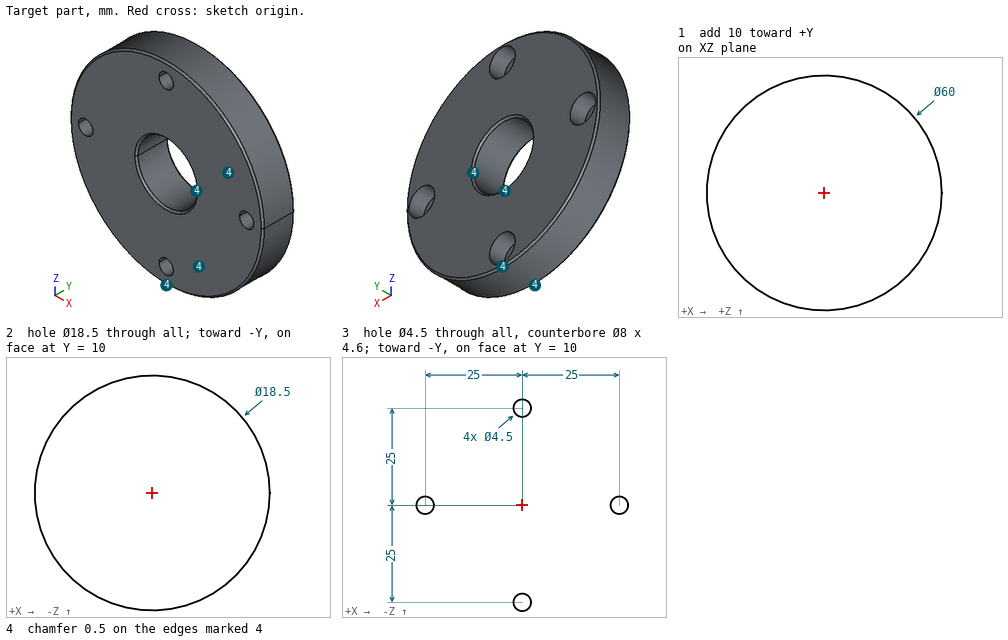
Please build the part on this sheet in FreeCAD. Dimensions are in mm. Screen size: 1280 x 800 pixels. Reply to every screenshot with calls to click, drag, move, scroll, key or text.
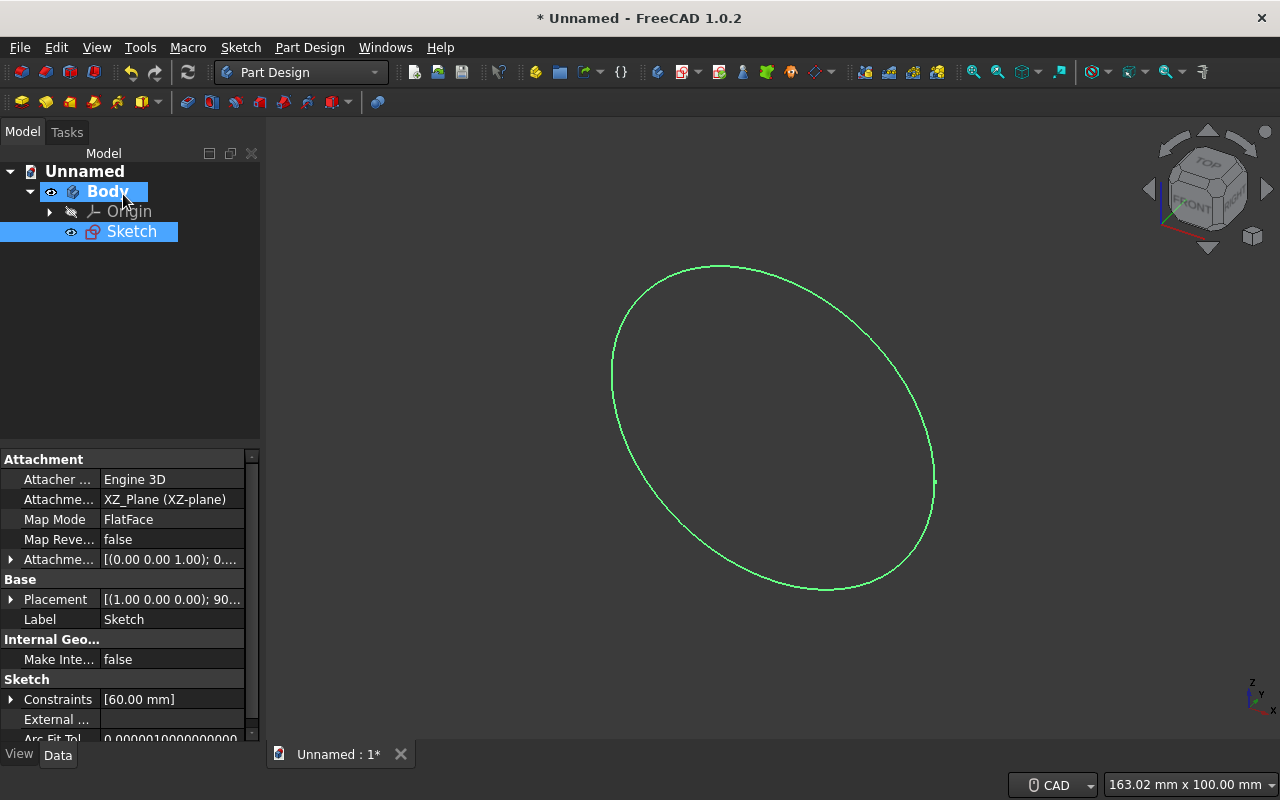
click(22, 102)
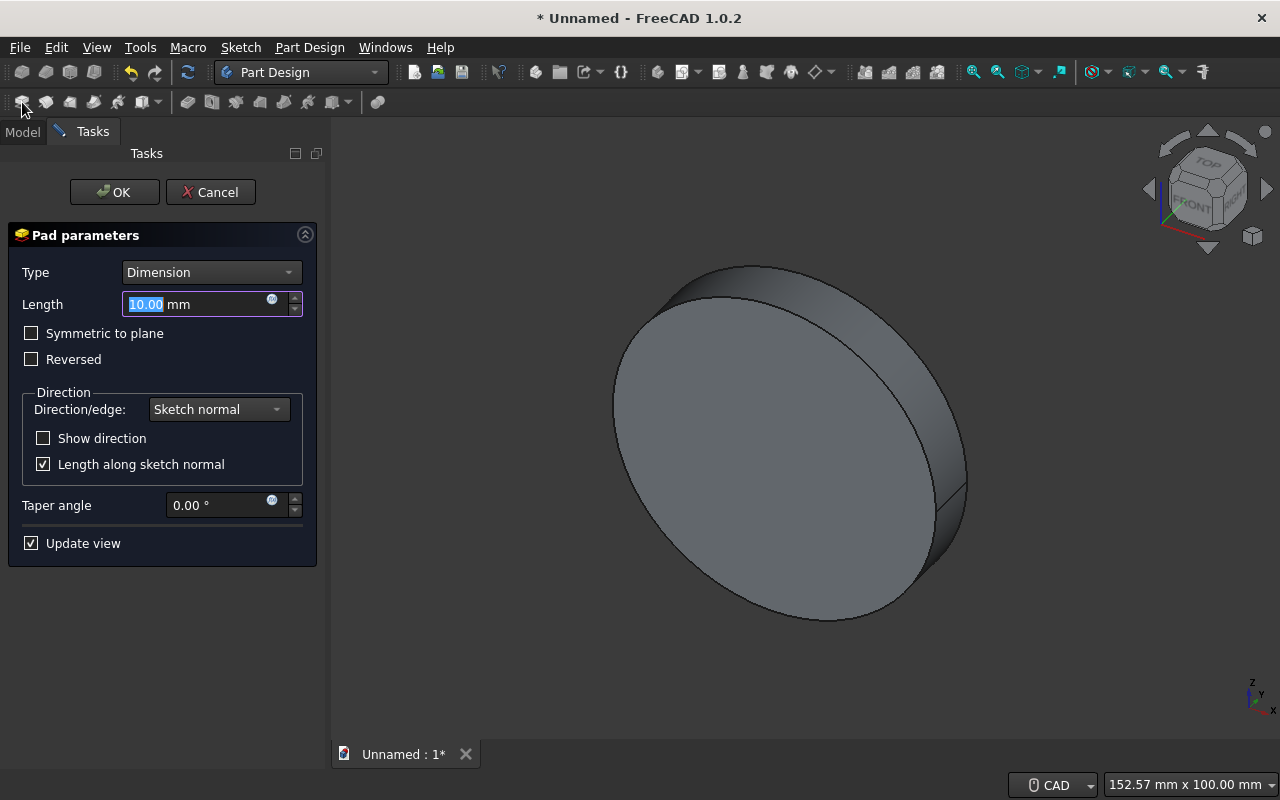
text(10)
key(Tab)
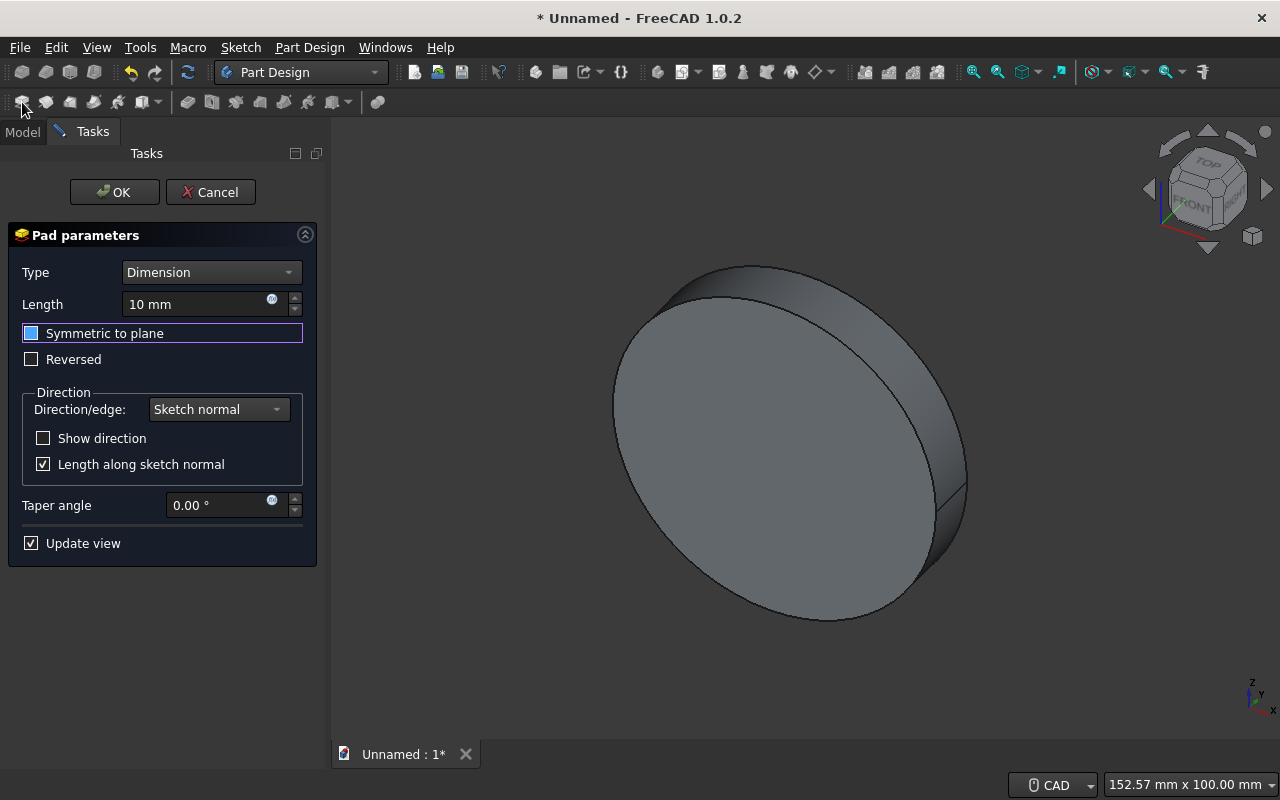
click(30, 359)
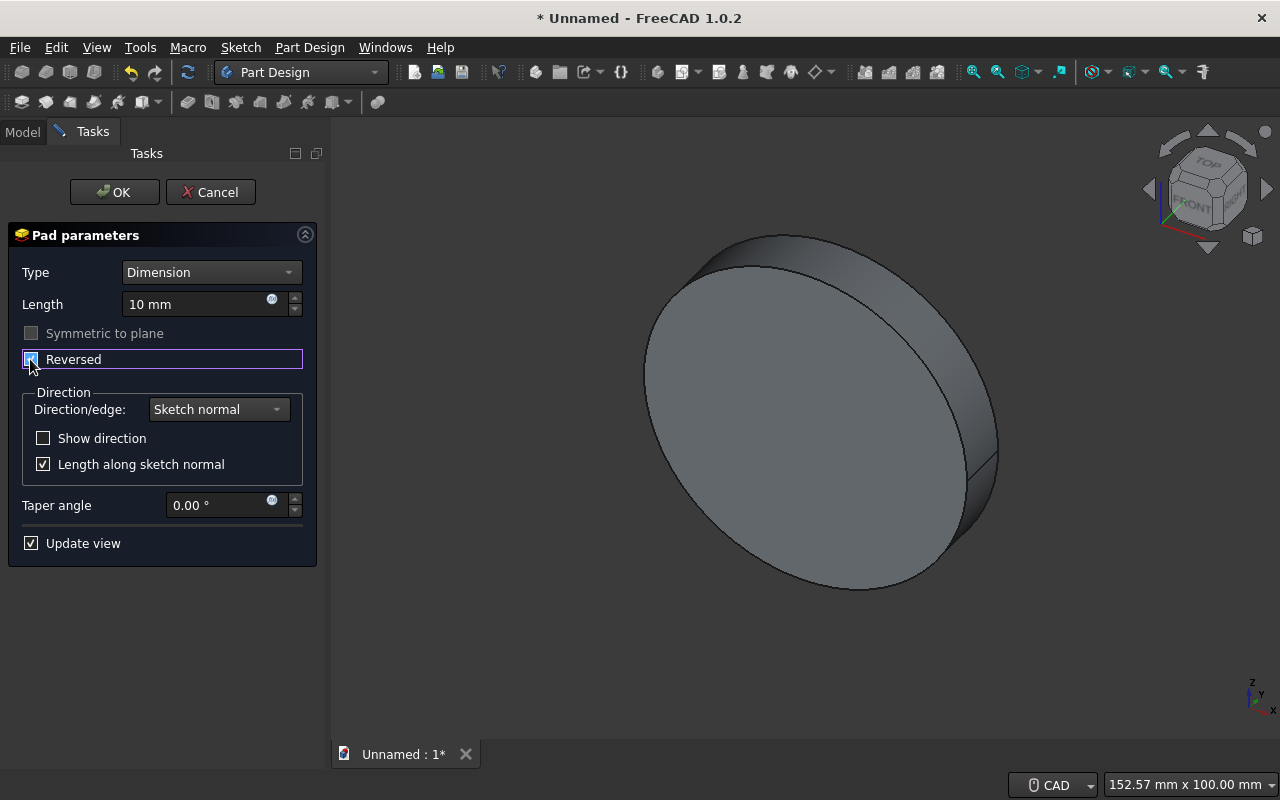
click(115, 192)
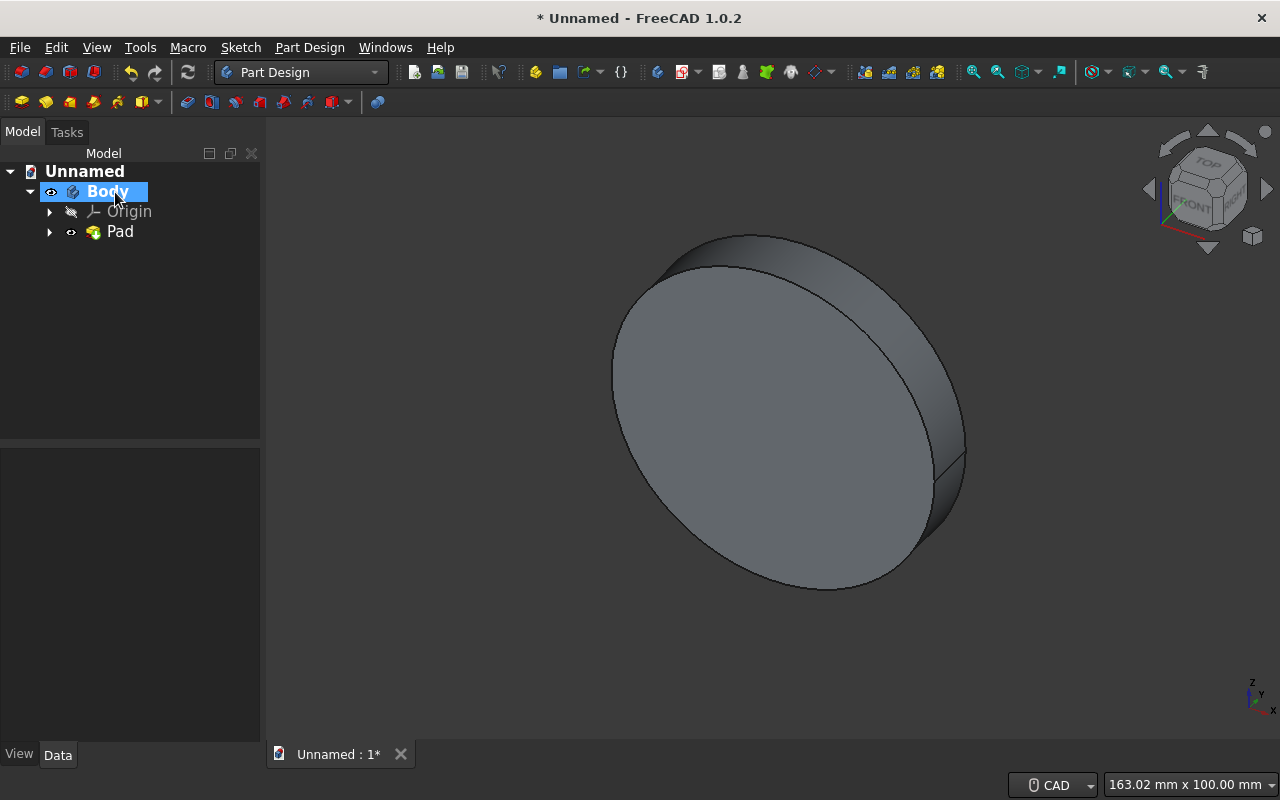
key(4)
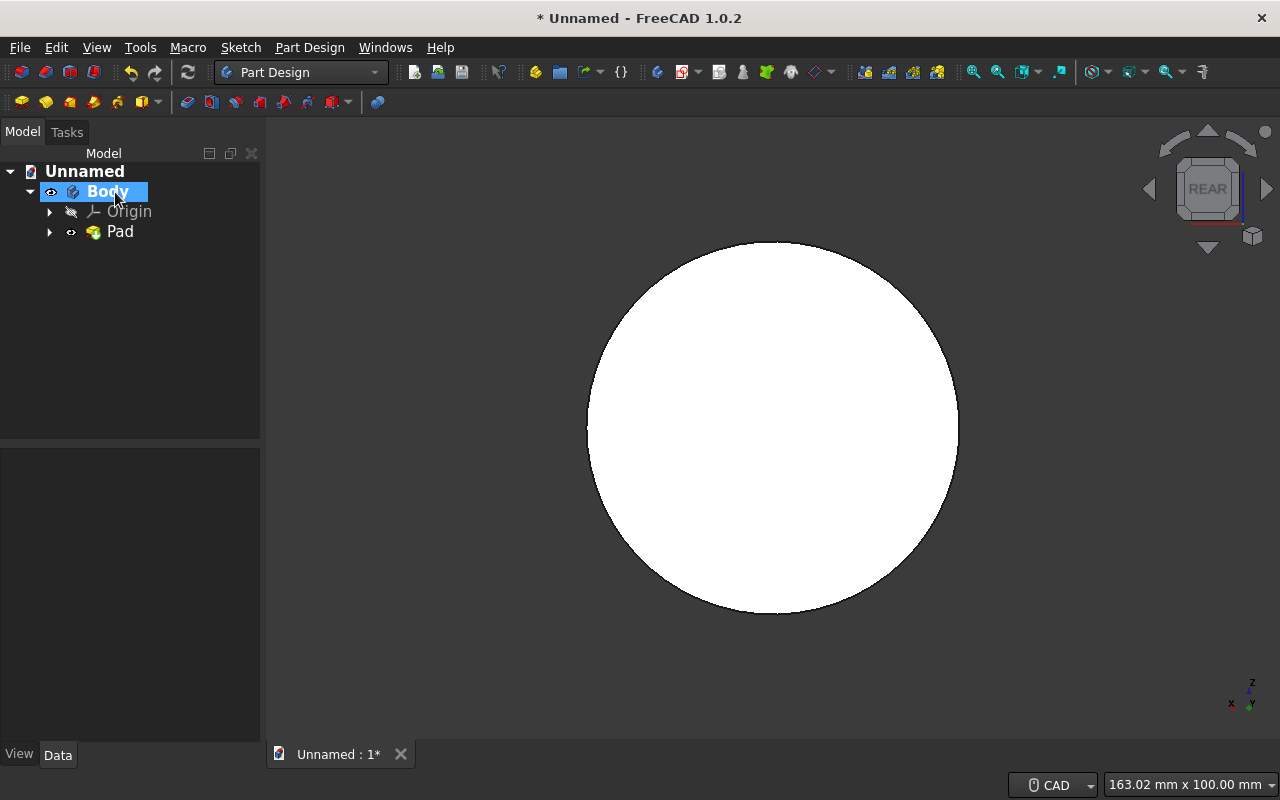
click(773, 427)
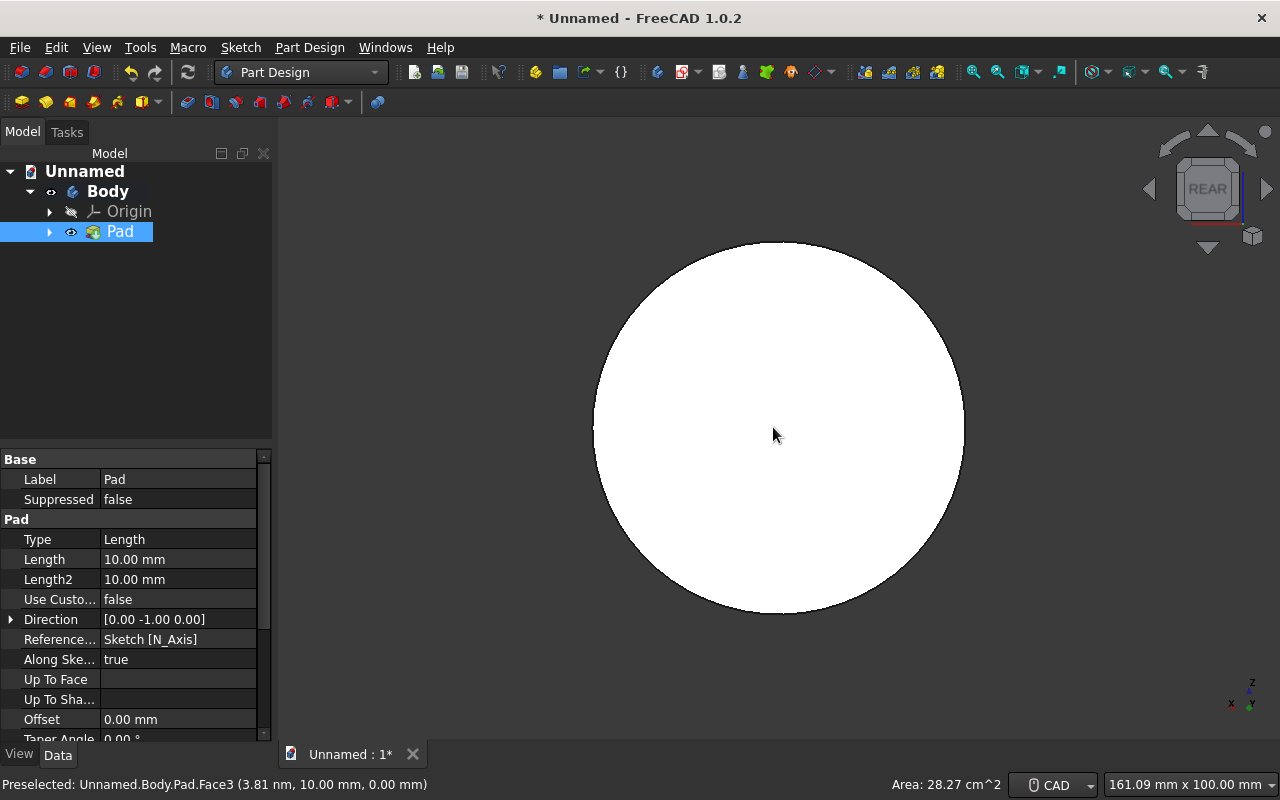
click(682, 72)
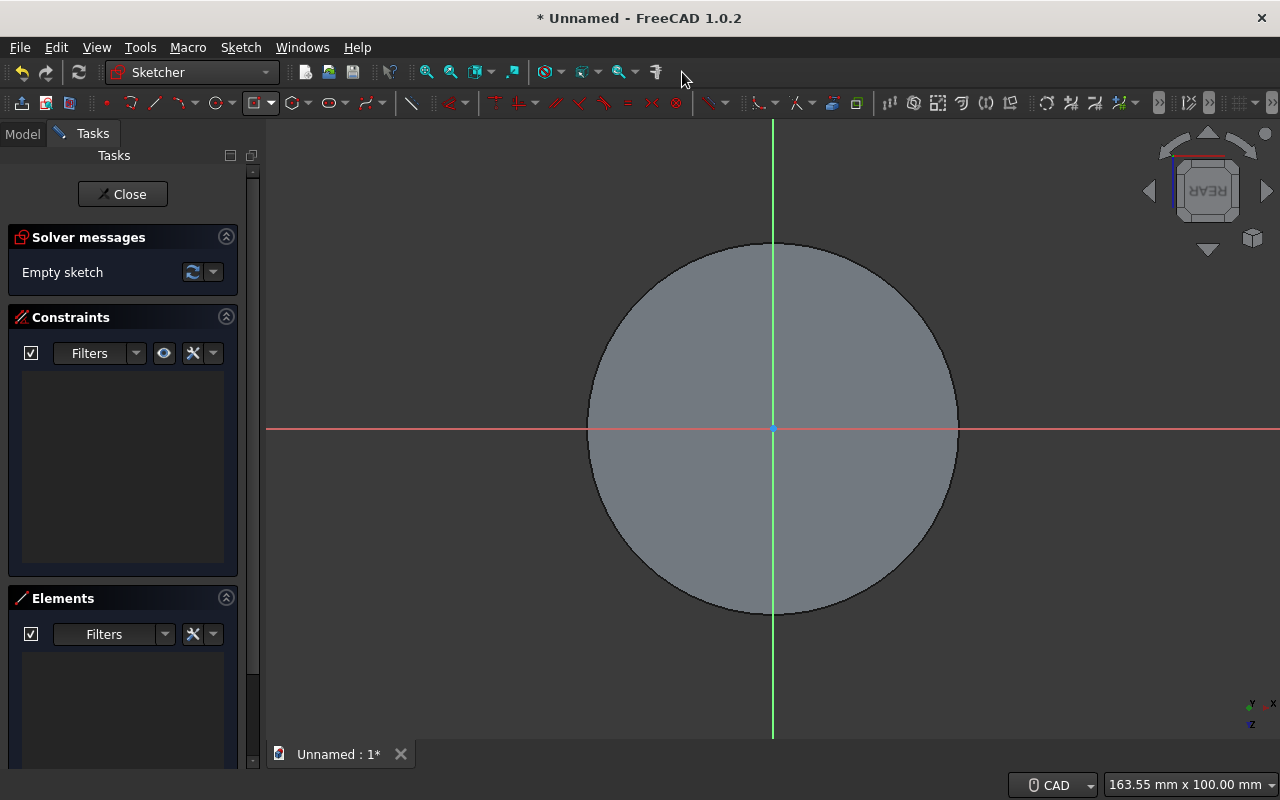
scroll(803, 429, up, 6)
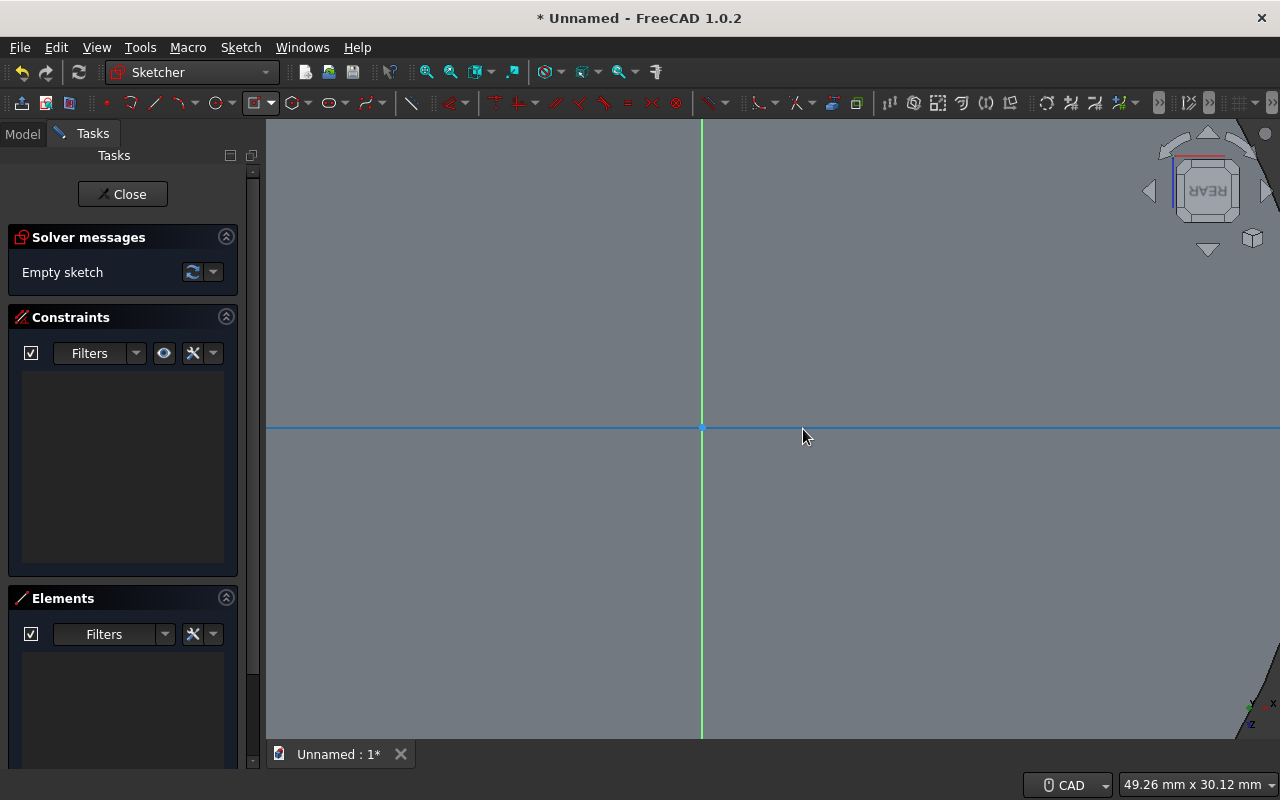
key(g)
key(c)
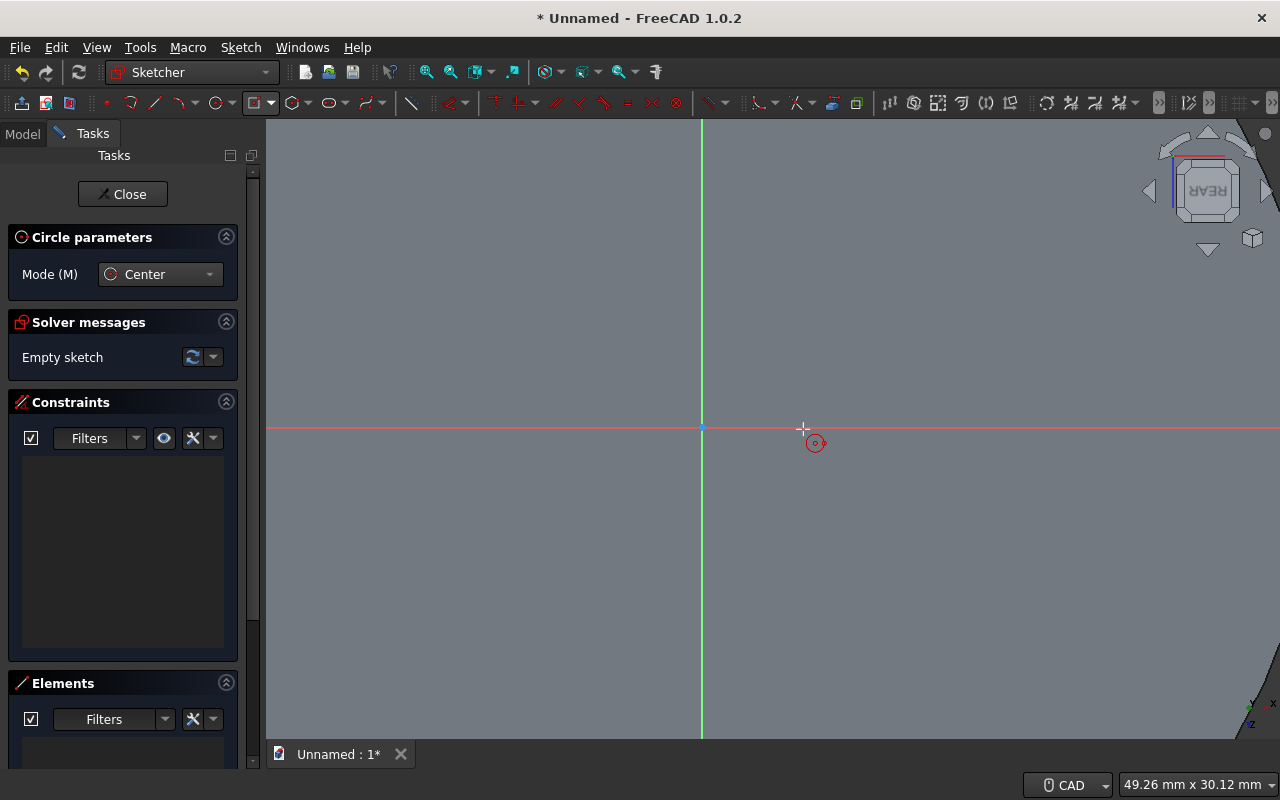
click(702, 428)
click(837, 293)
key(Escape)